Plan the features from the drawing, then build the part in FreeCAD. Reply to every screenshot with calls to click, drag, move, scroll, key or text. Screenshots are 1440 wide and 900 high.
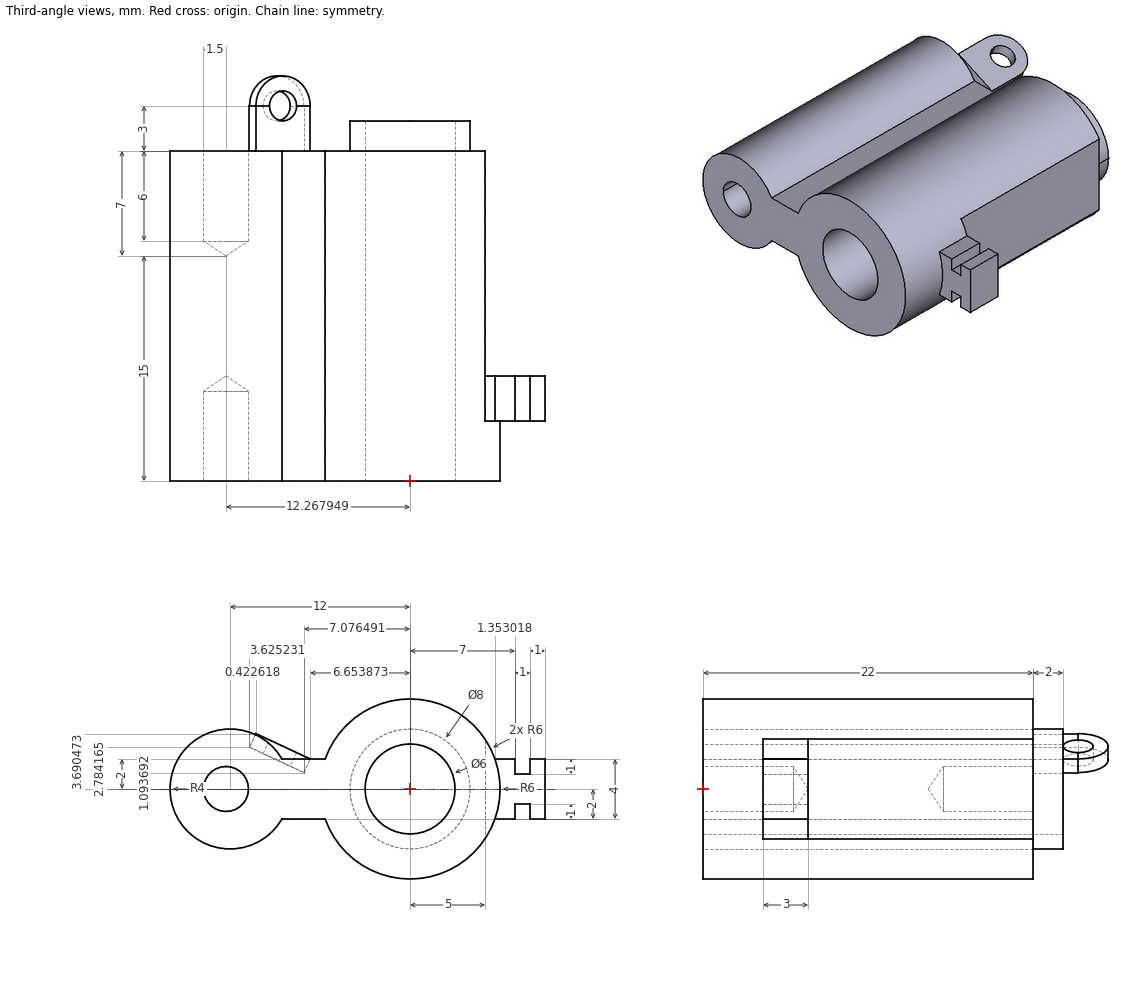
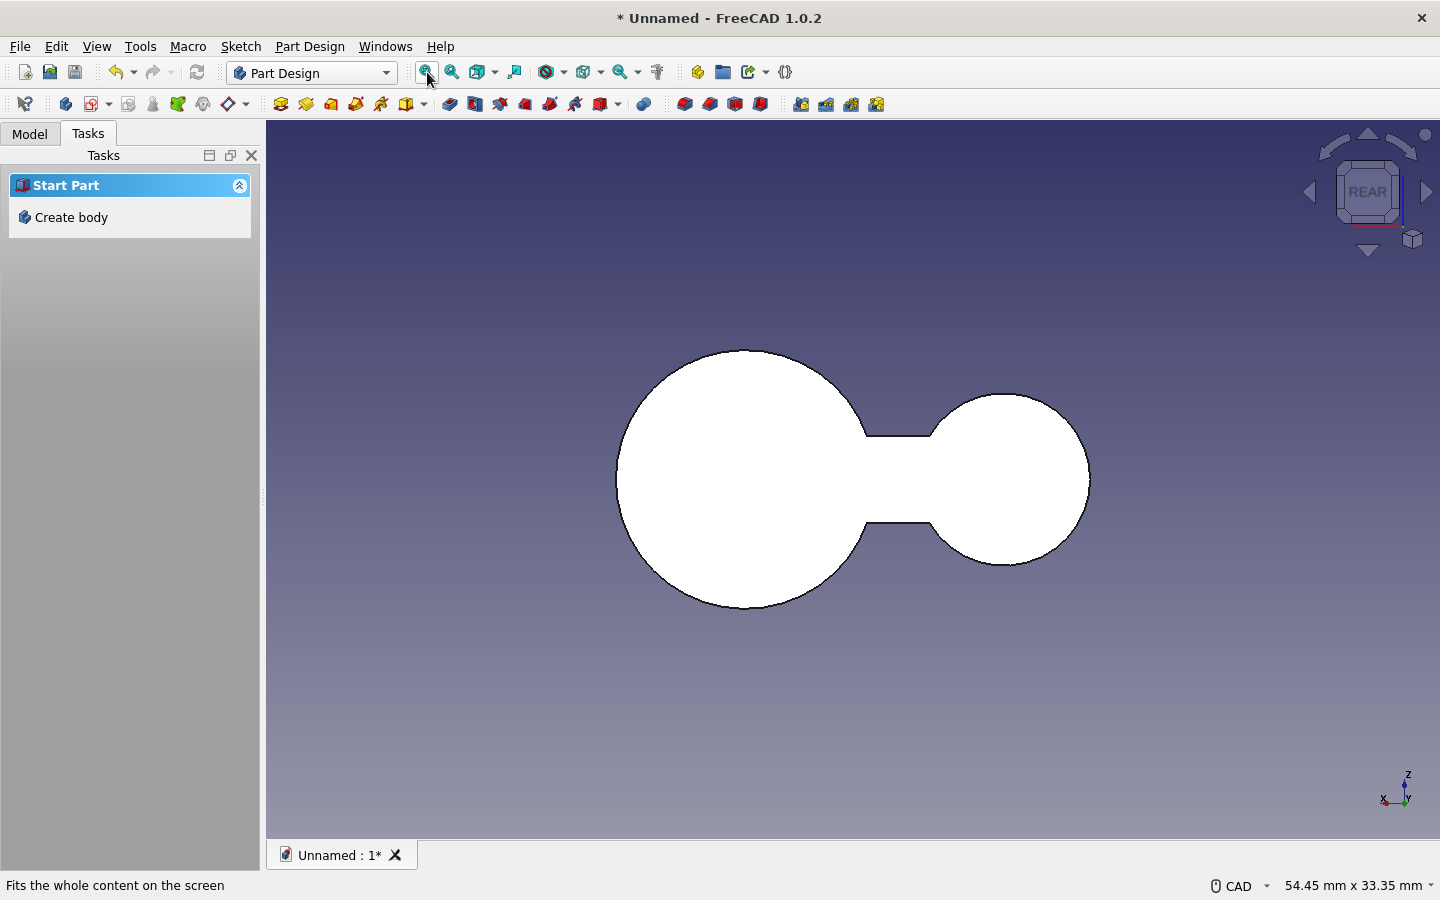
click(427, 72)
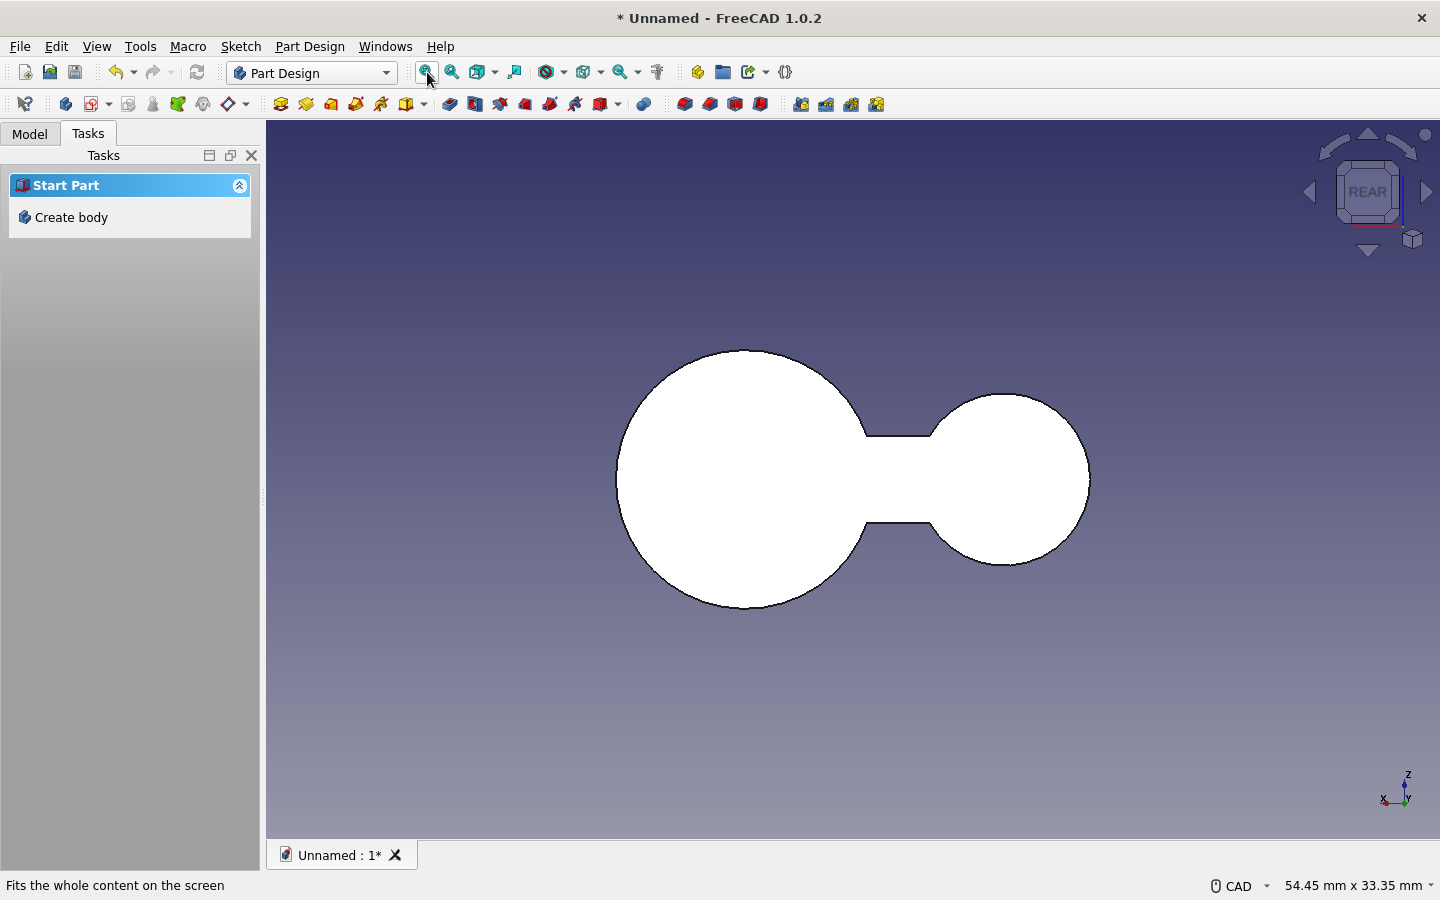
click(717, 479)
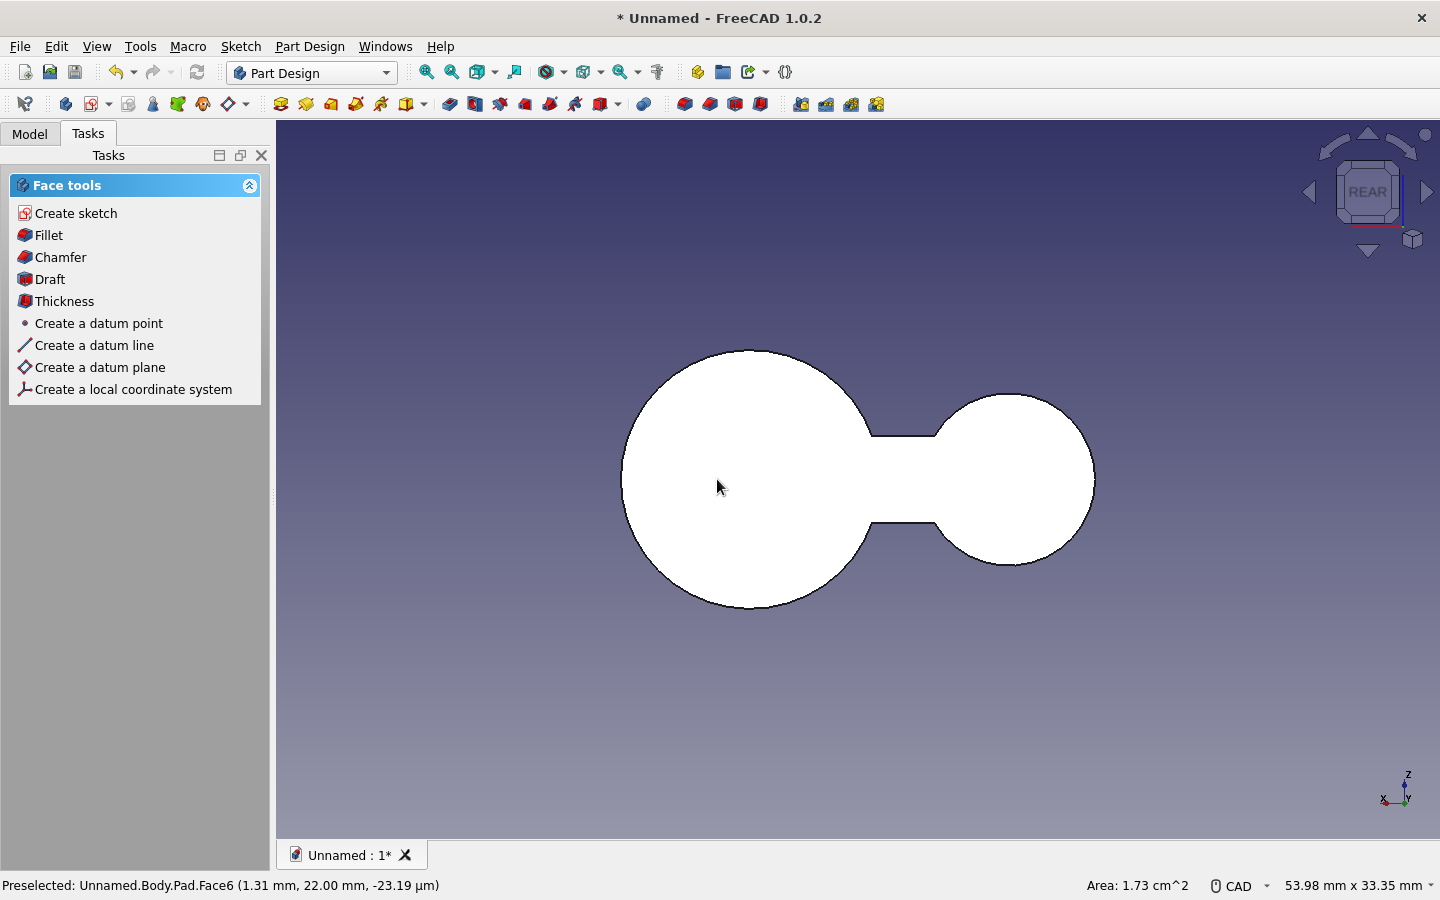
click(90, 104)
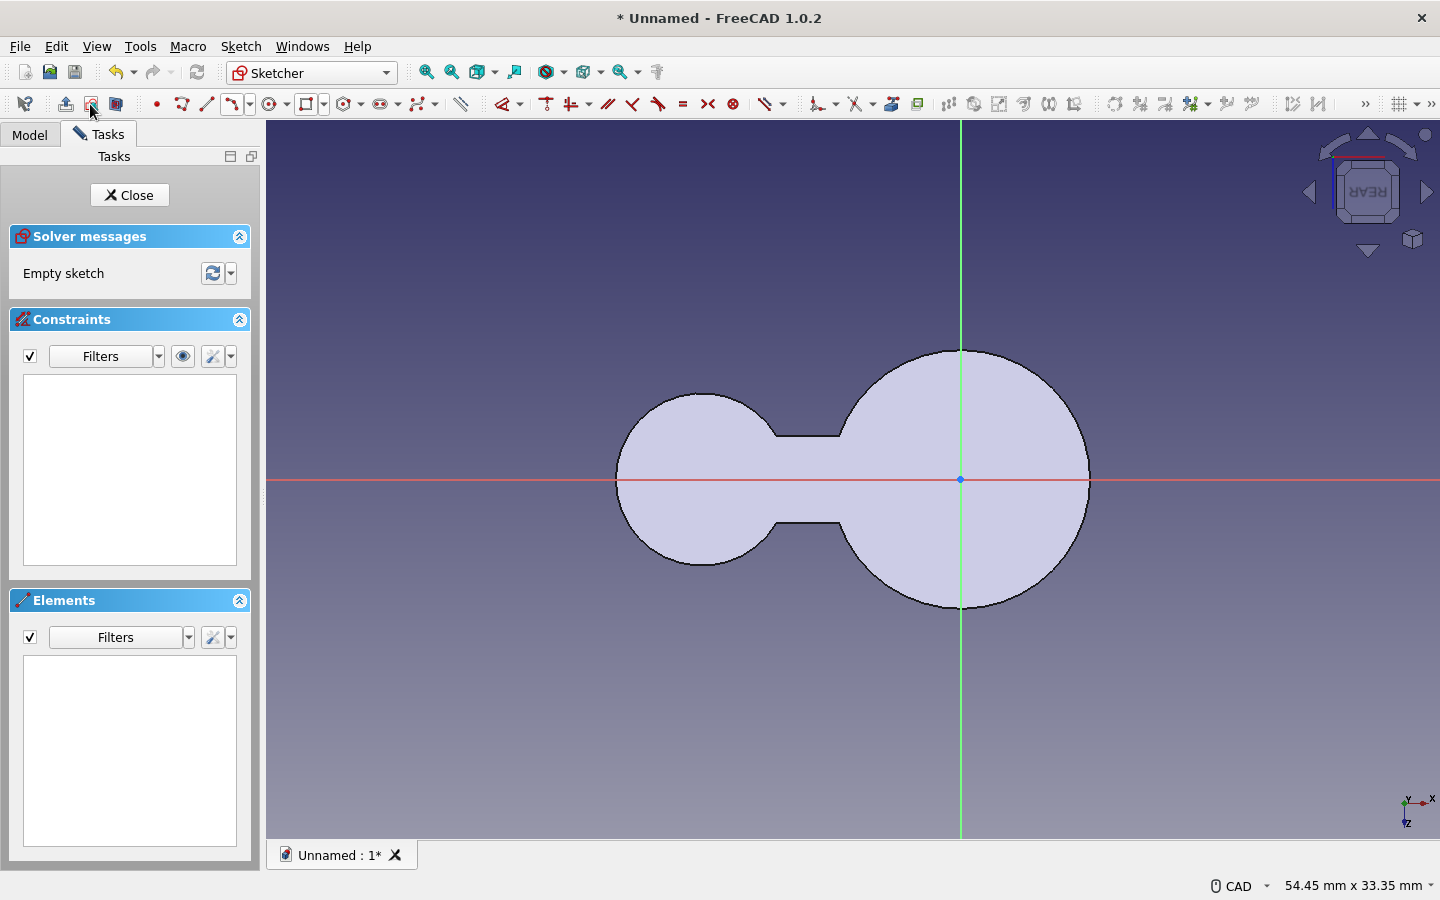
scroll(772, 539, up, 10)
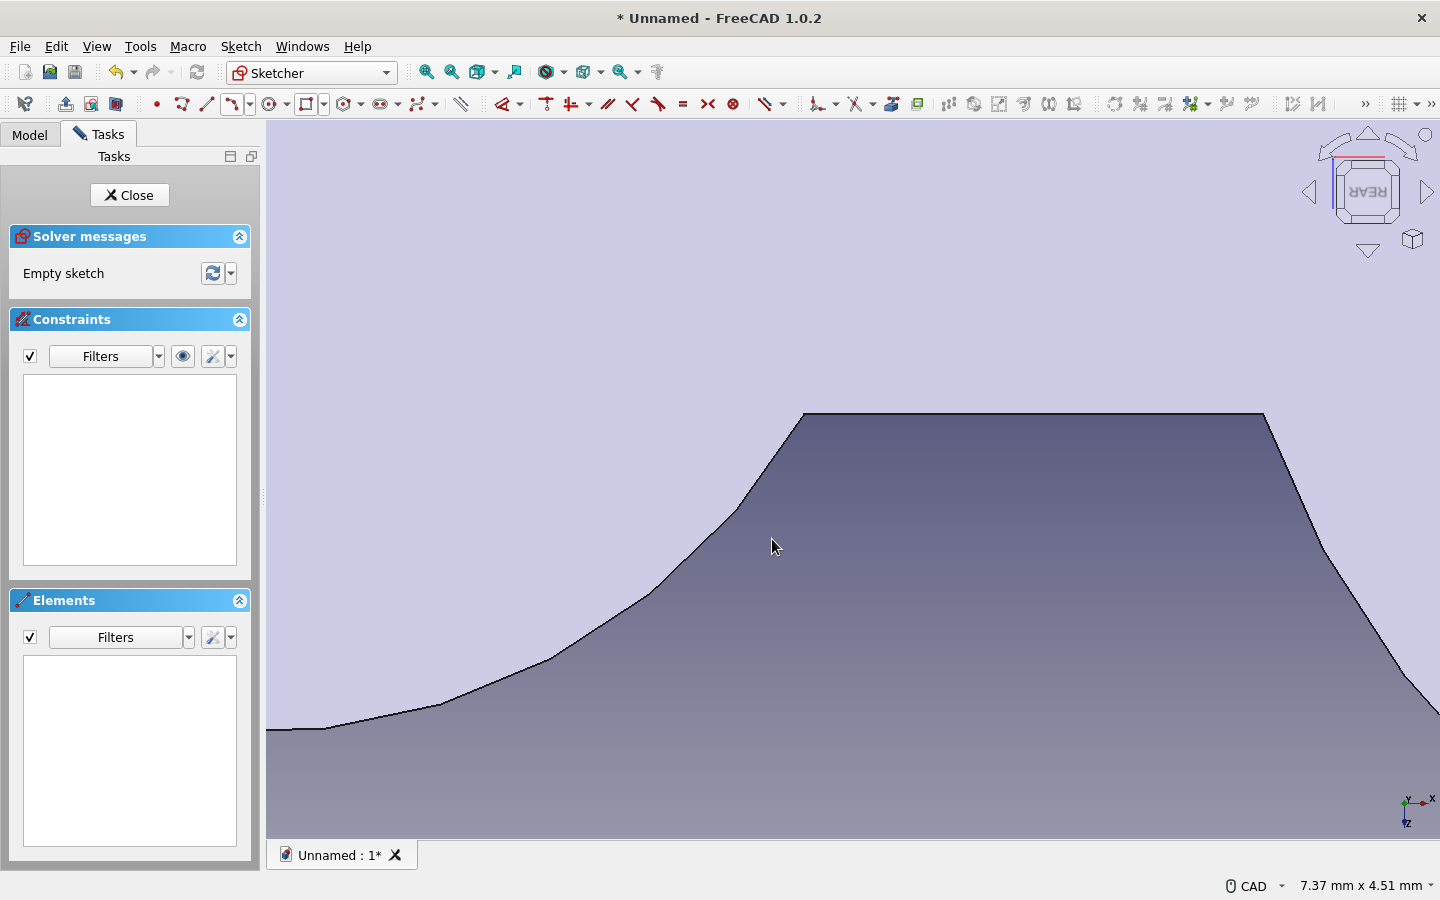
click(182, 104)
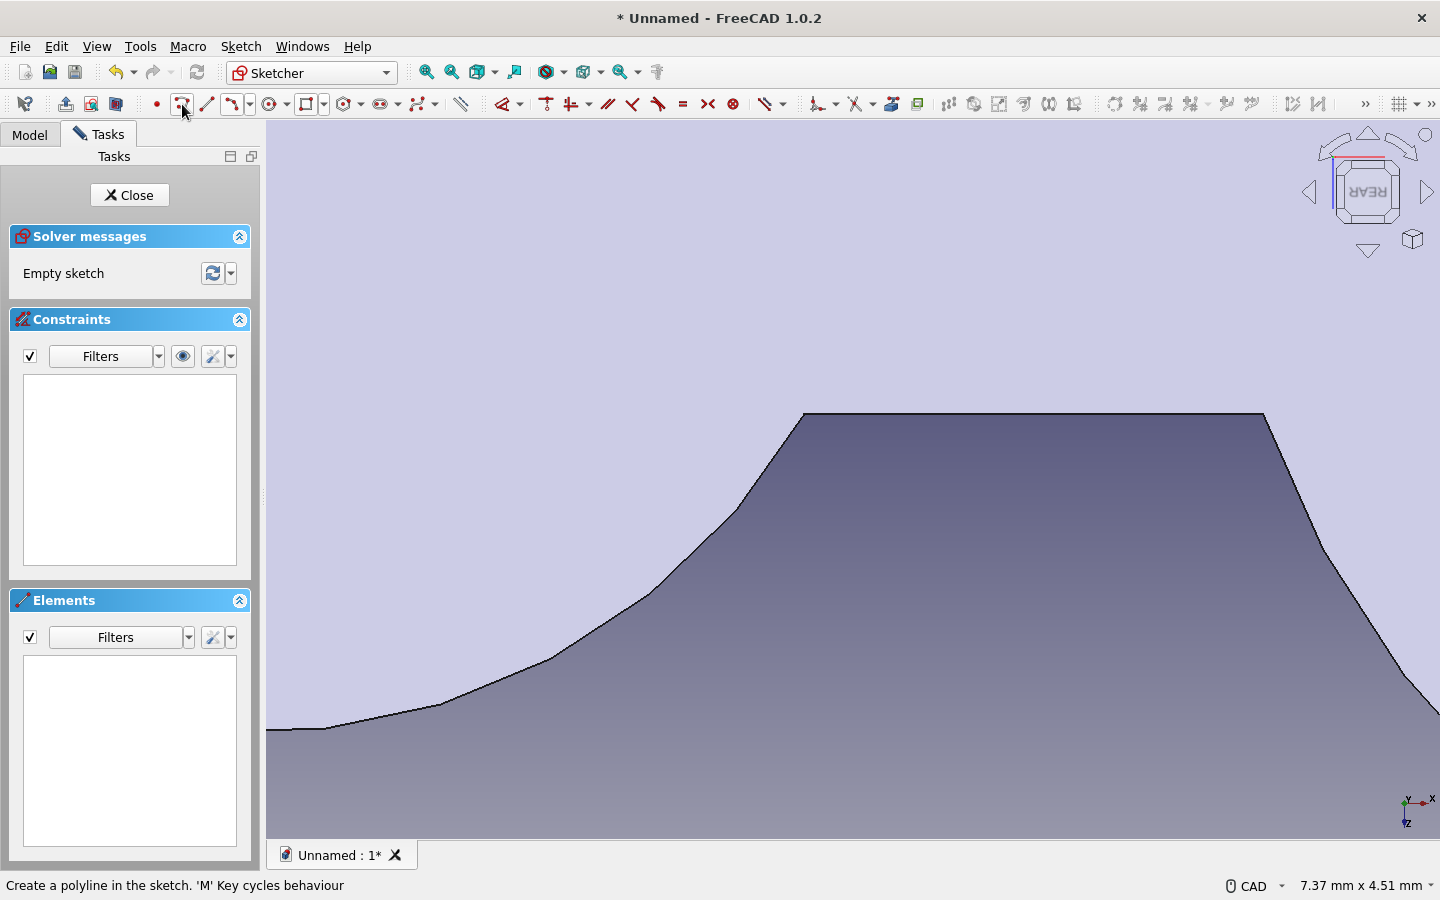
click(1104, 414)
click(1037, 270)
click(459, 539)
click(527, 684)
click(1104, 415)
key(Escape)
key(Escape)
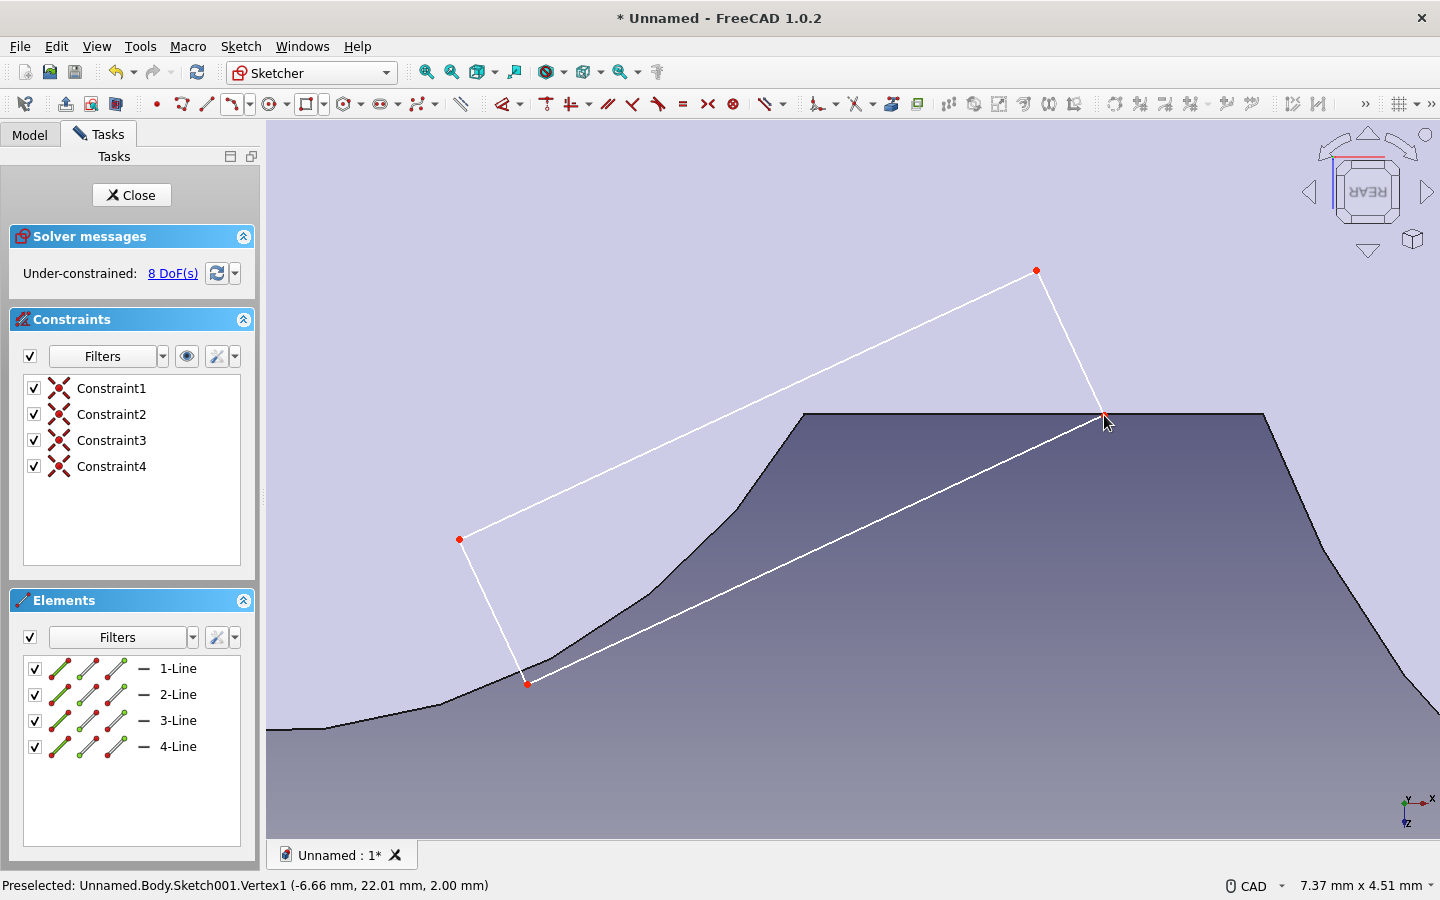
click(502, 104)